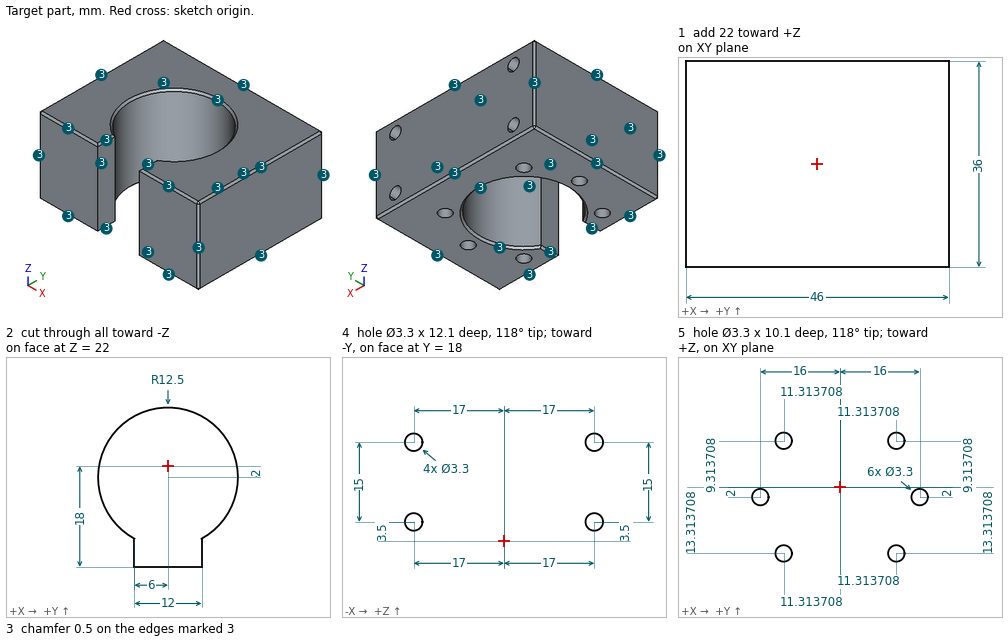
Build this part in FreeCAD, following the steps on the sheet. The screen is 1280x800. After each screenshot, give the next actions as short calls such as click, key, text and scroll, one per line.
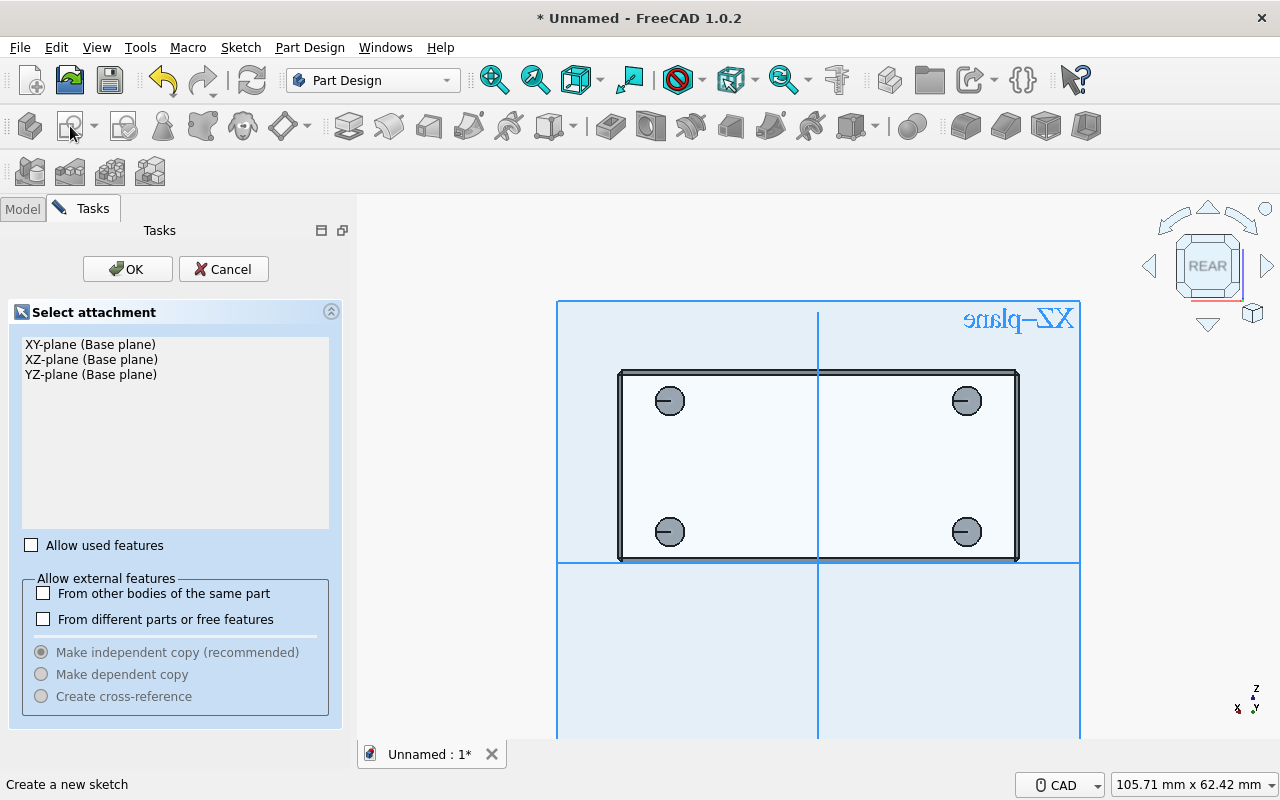
click(82, 344)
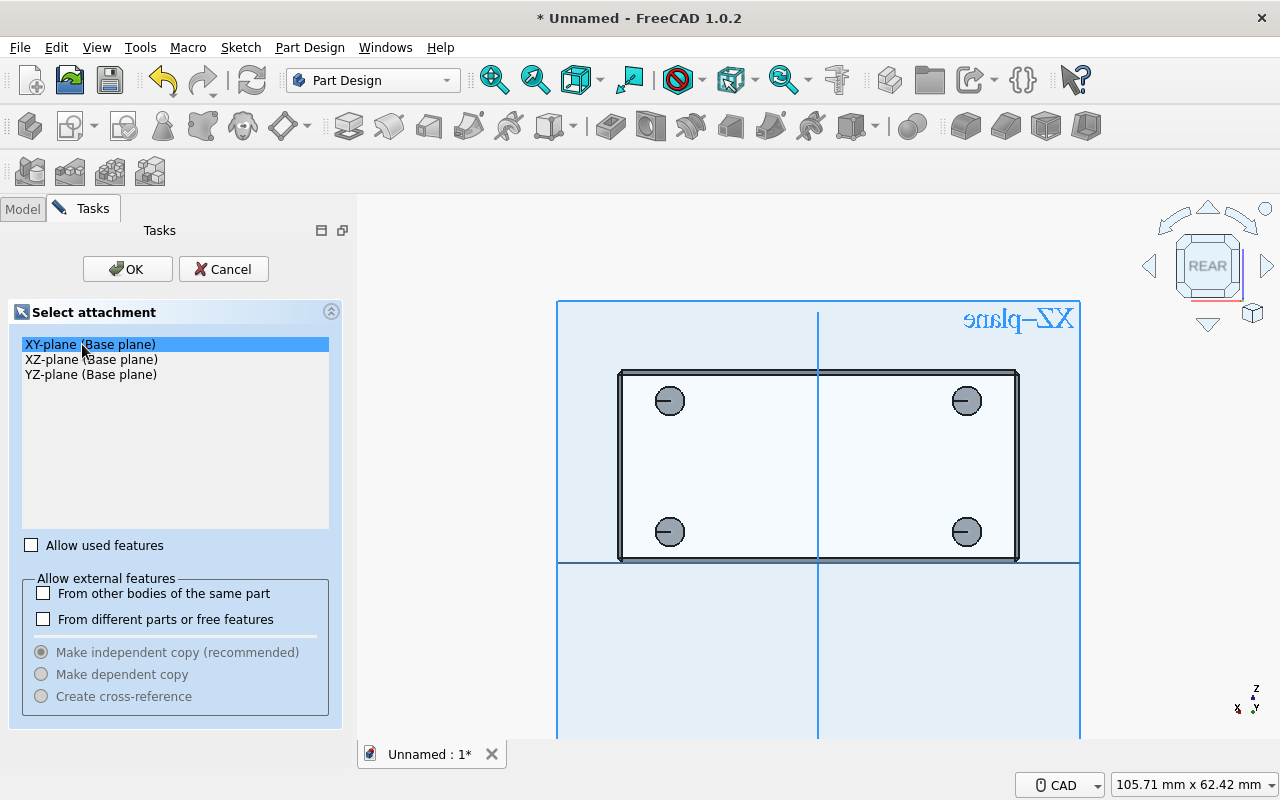
click(128, 269)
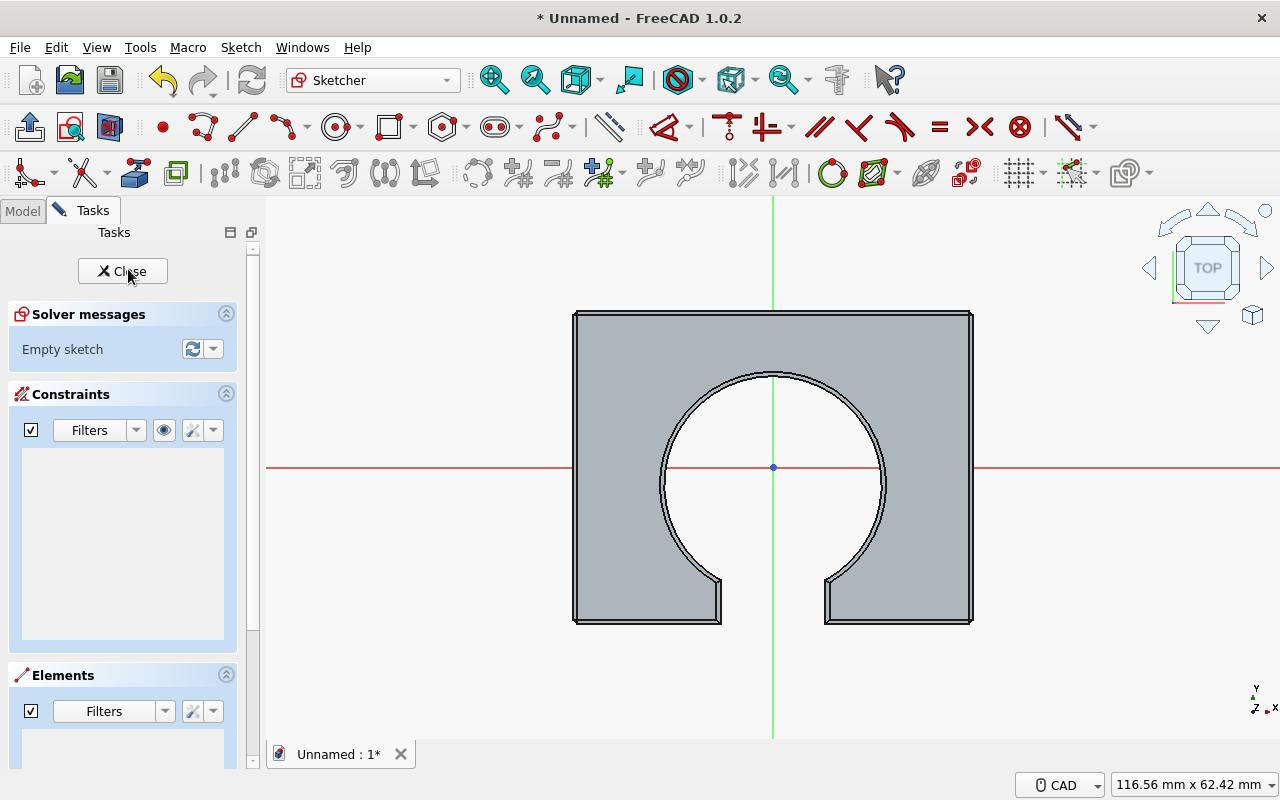
click(110, 128)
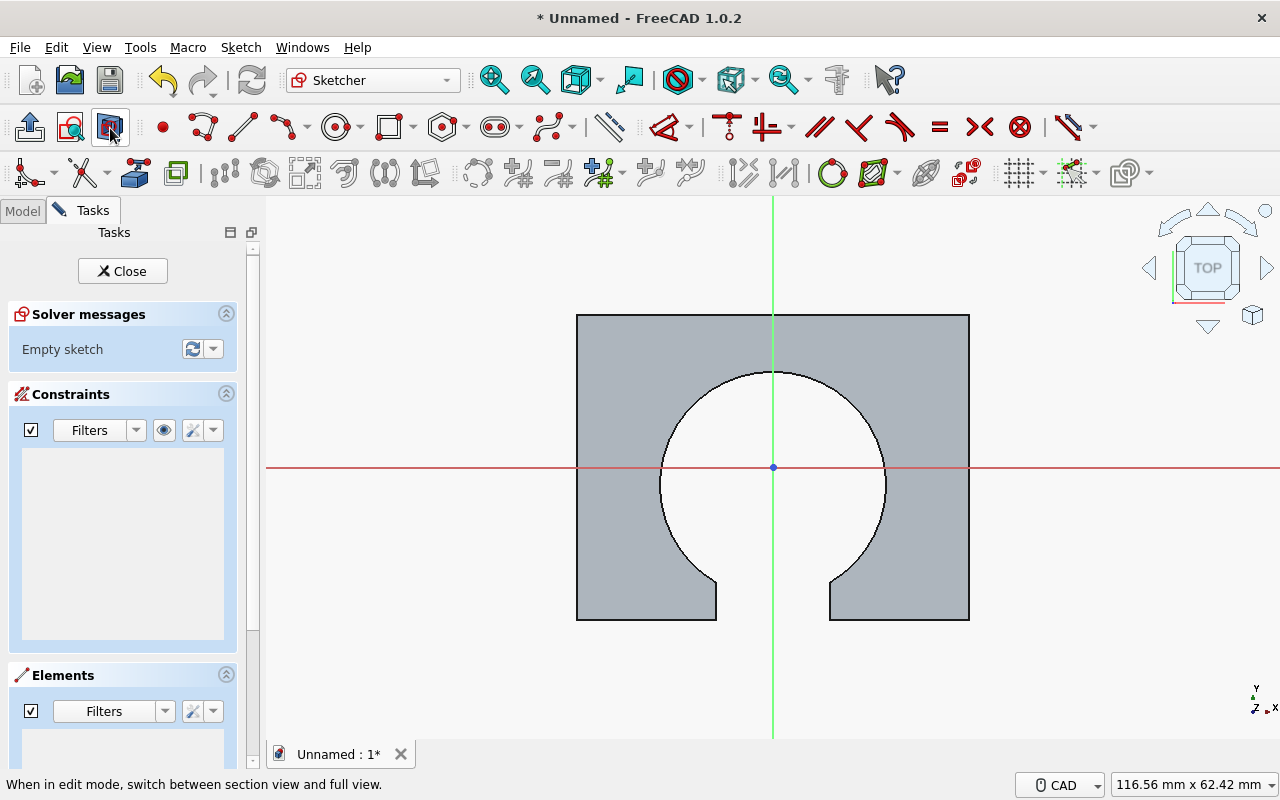
scroll(912, 520, up, 2)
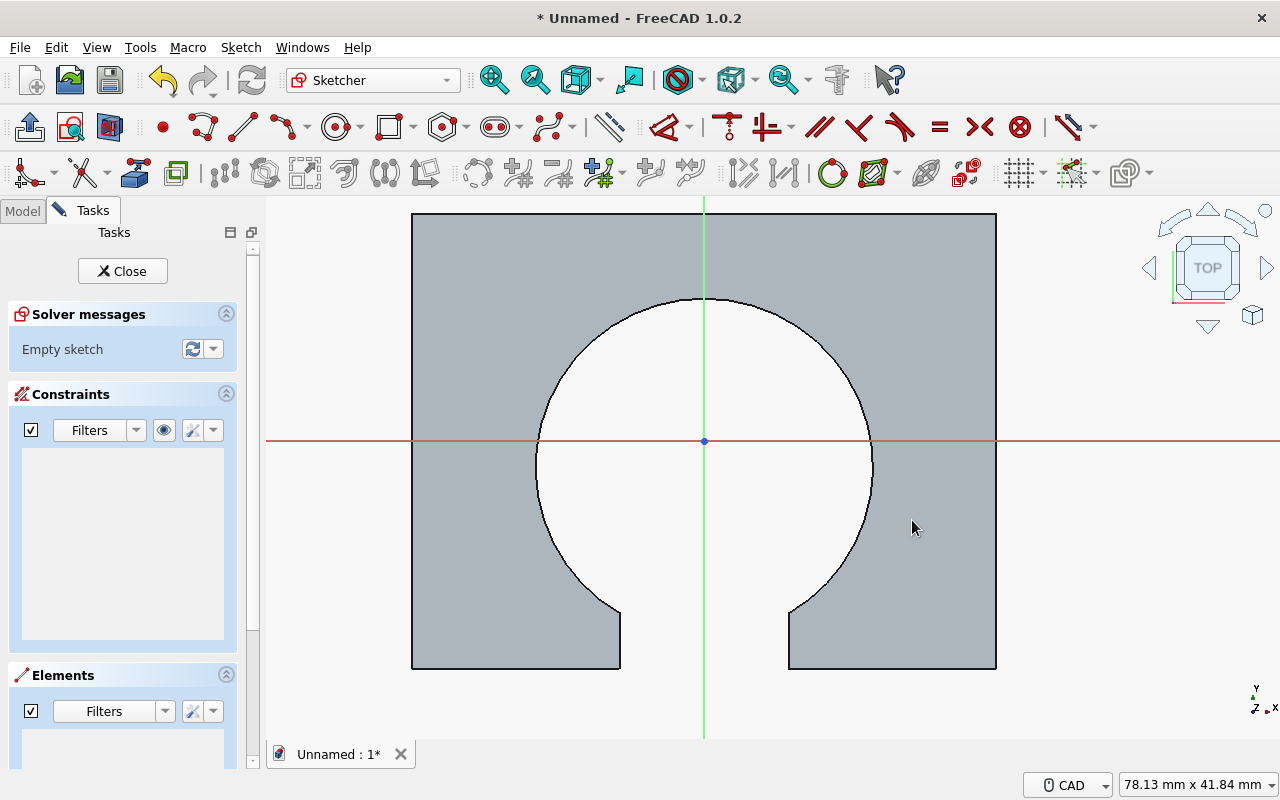
click(336, 128)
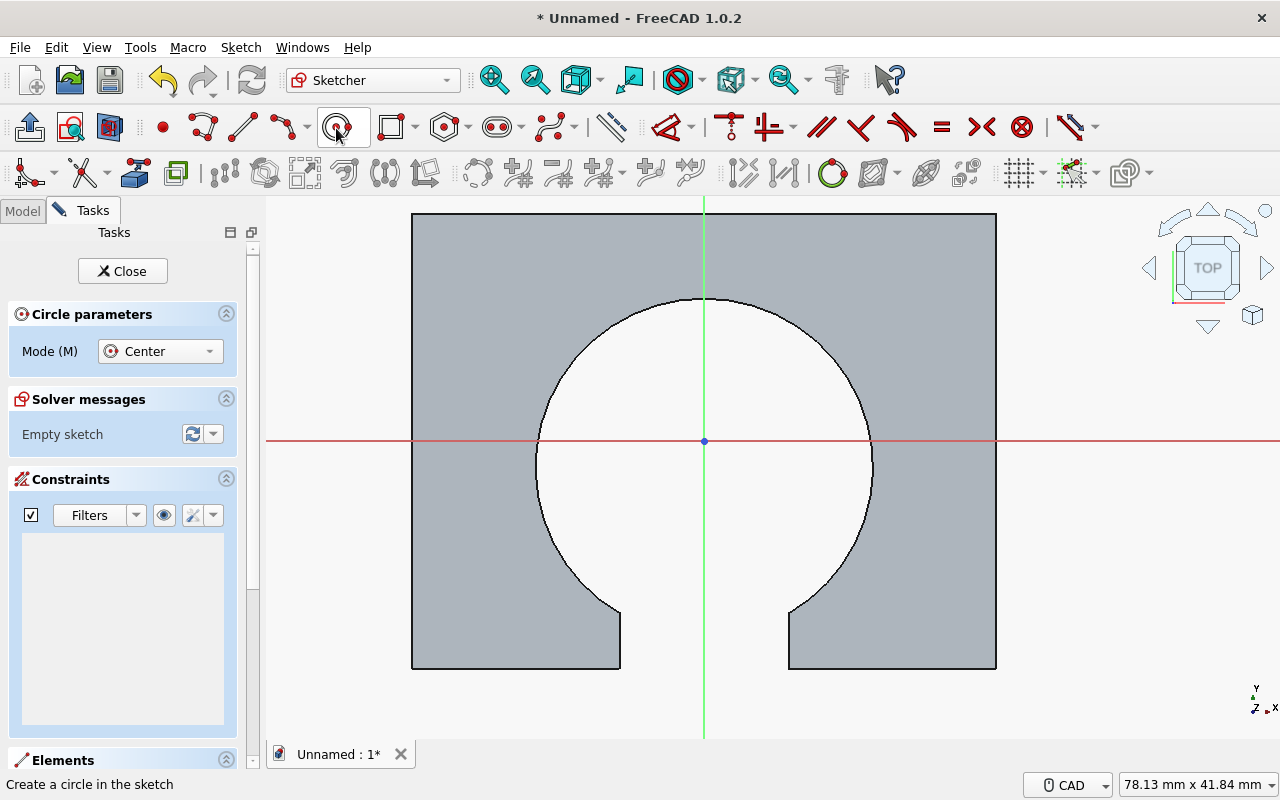
click(912, 467)
move(927, 482)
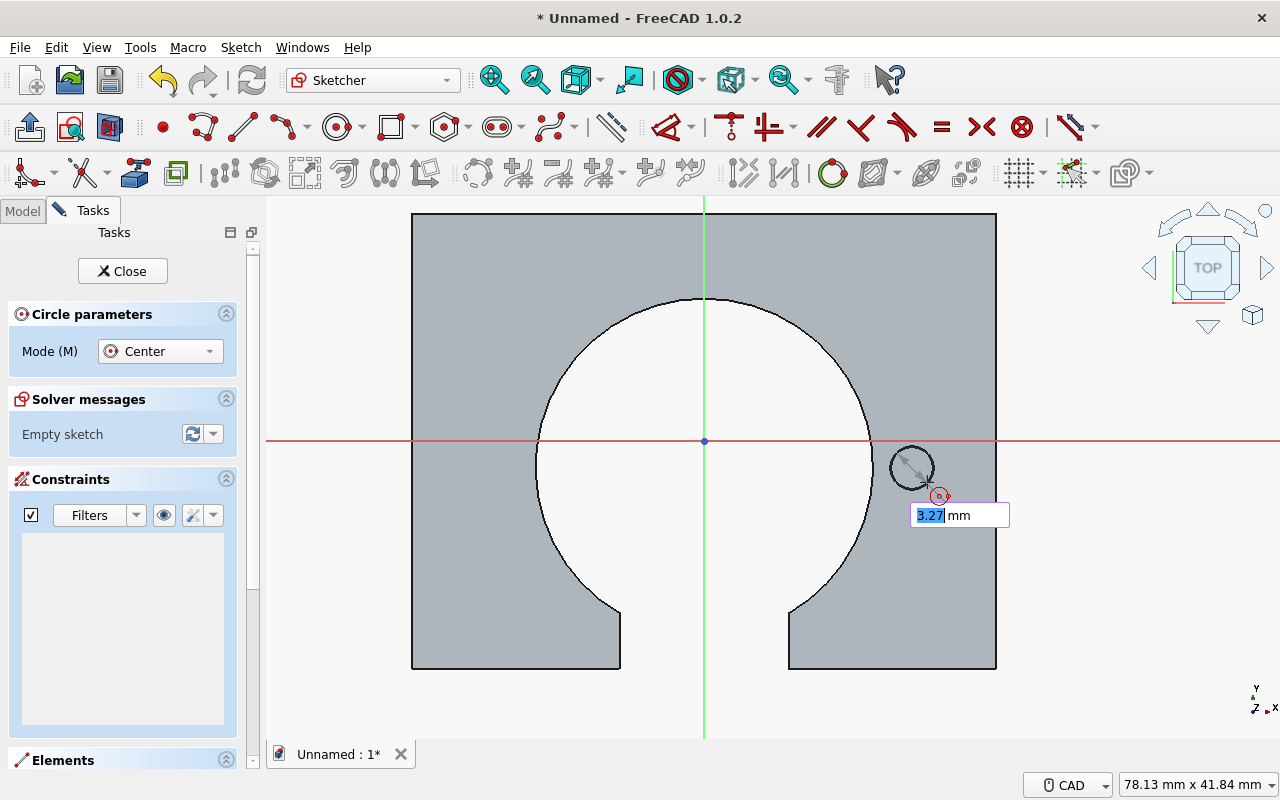
text(3.3)
key(Return)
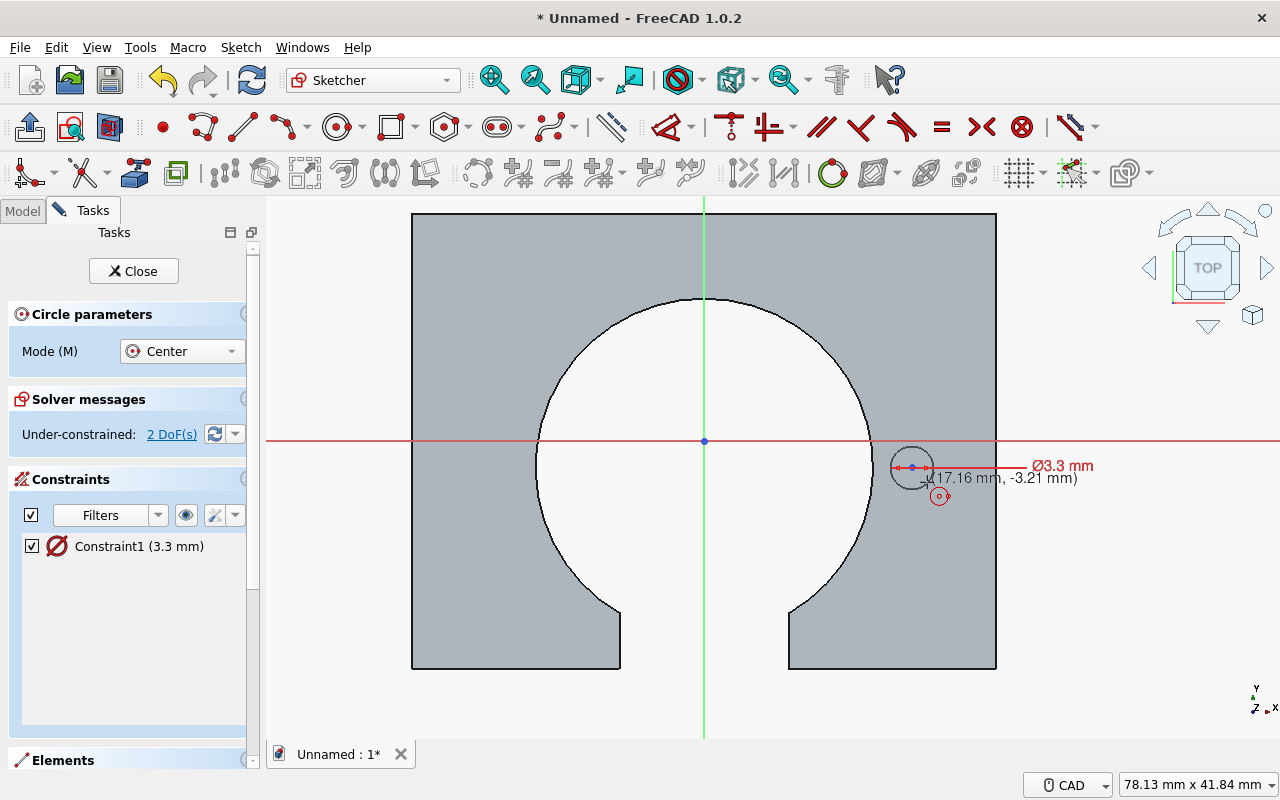
click(851, 321)
move(866, 305)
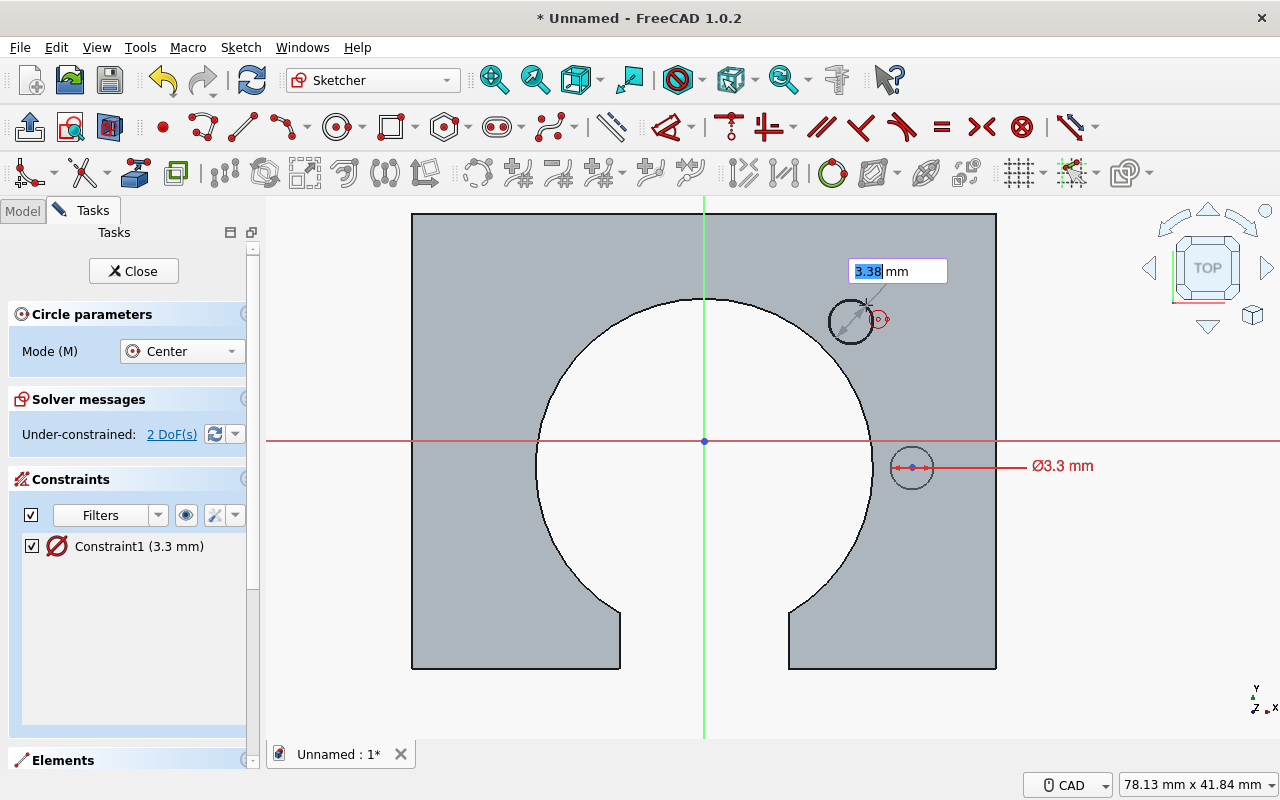
text(3.3)
key(Return)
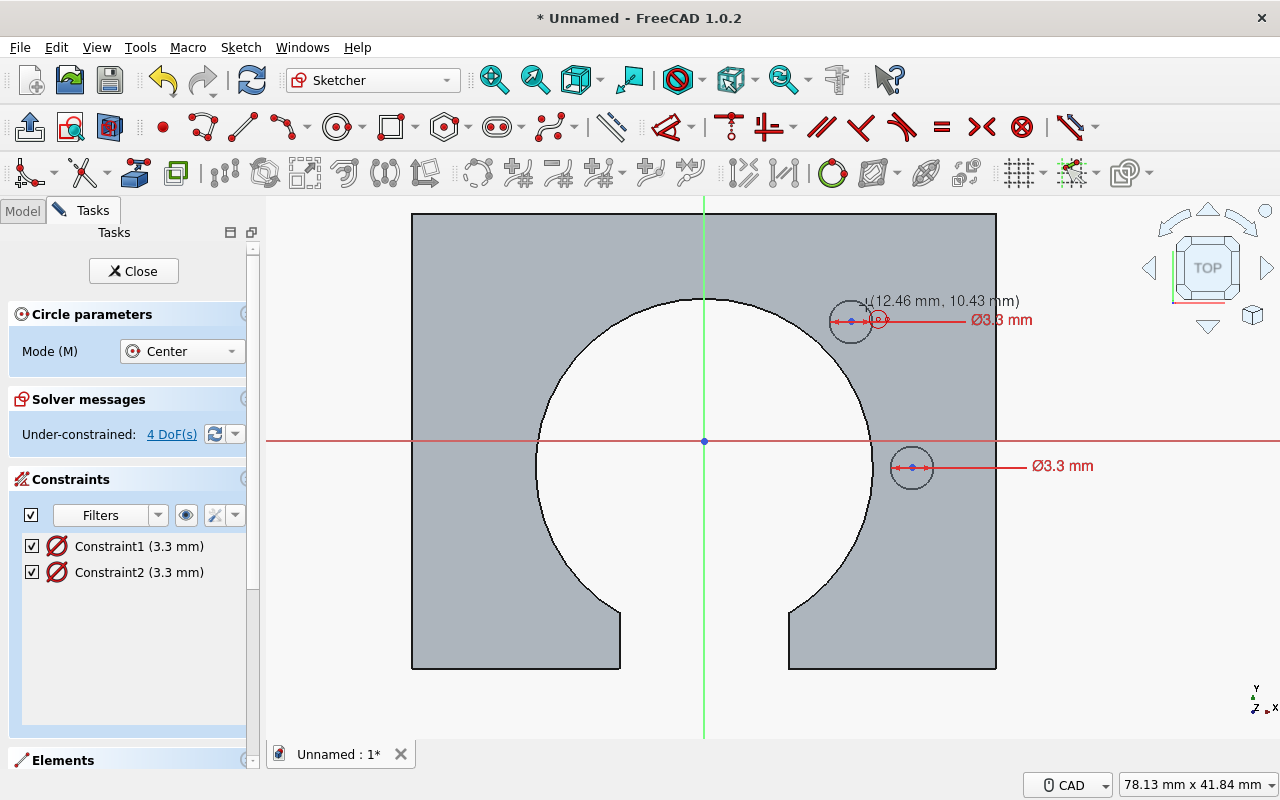
click(557, 321)
move(573, 305)